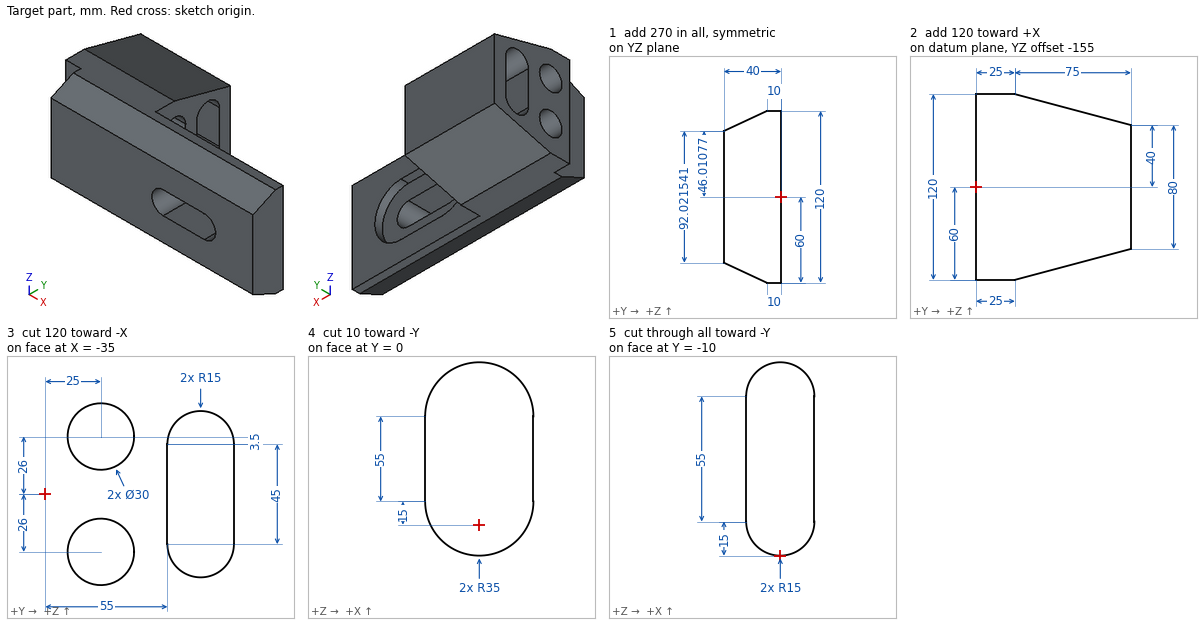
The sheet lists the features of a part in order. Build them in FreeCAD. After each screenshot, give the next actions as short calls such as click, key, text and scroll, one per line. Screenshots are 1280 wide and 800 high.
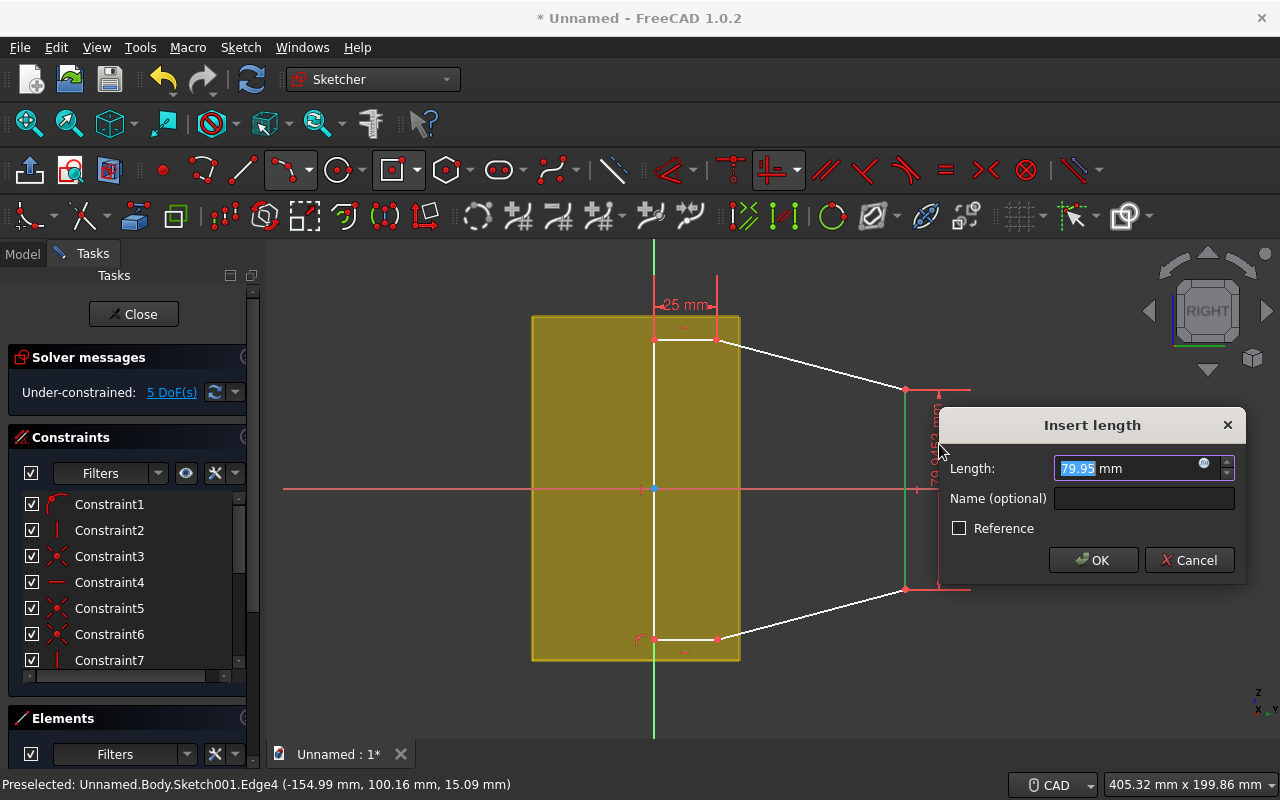
text(80)
key(Return)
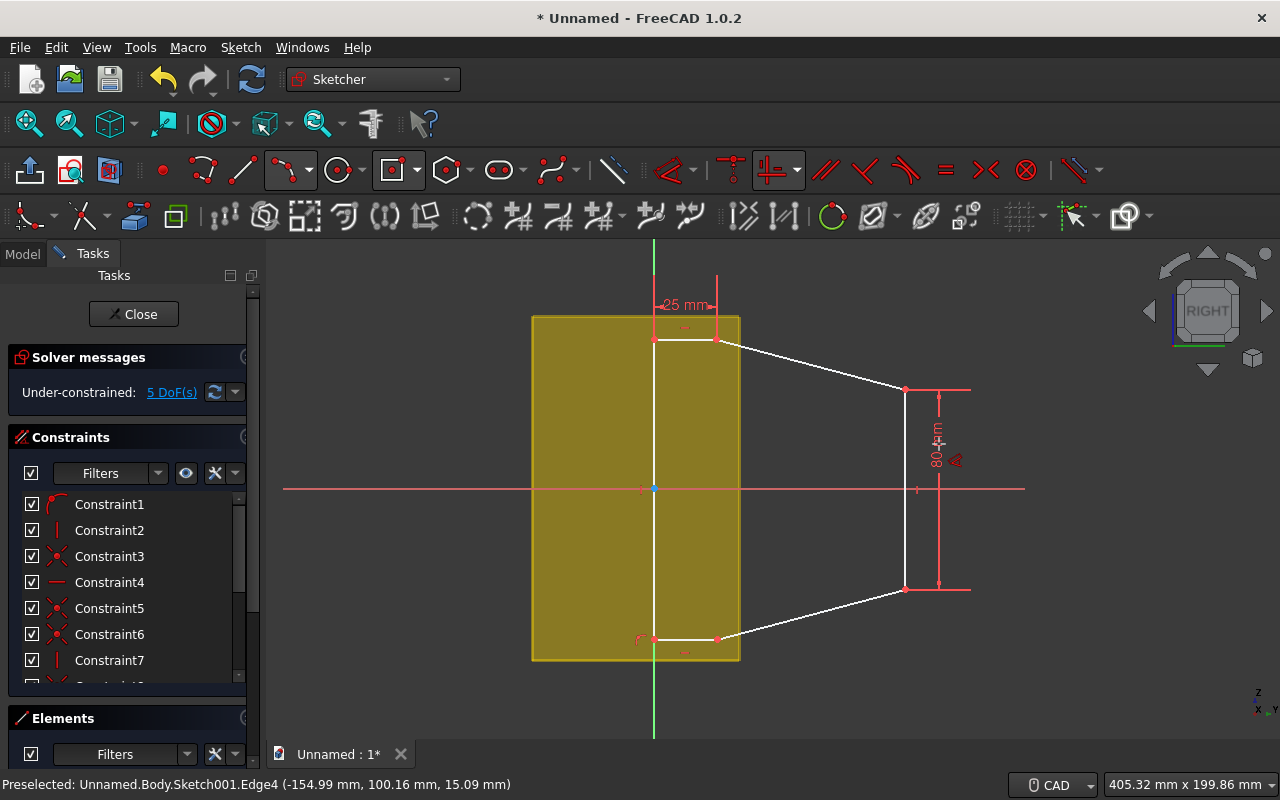
click(698, 640)
click(686, 674)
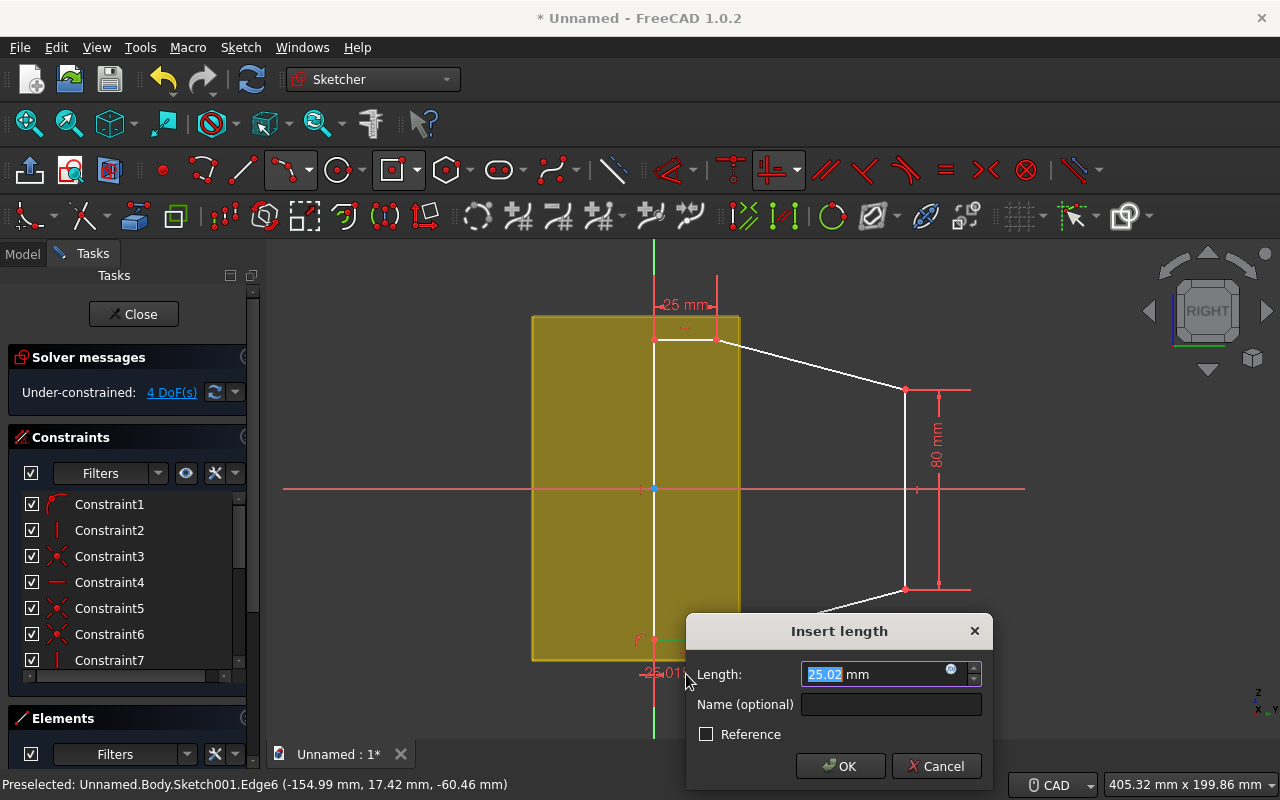
text(25)
key(Return)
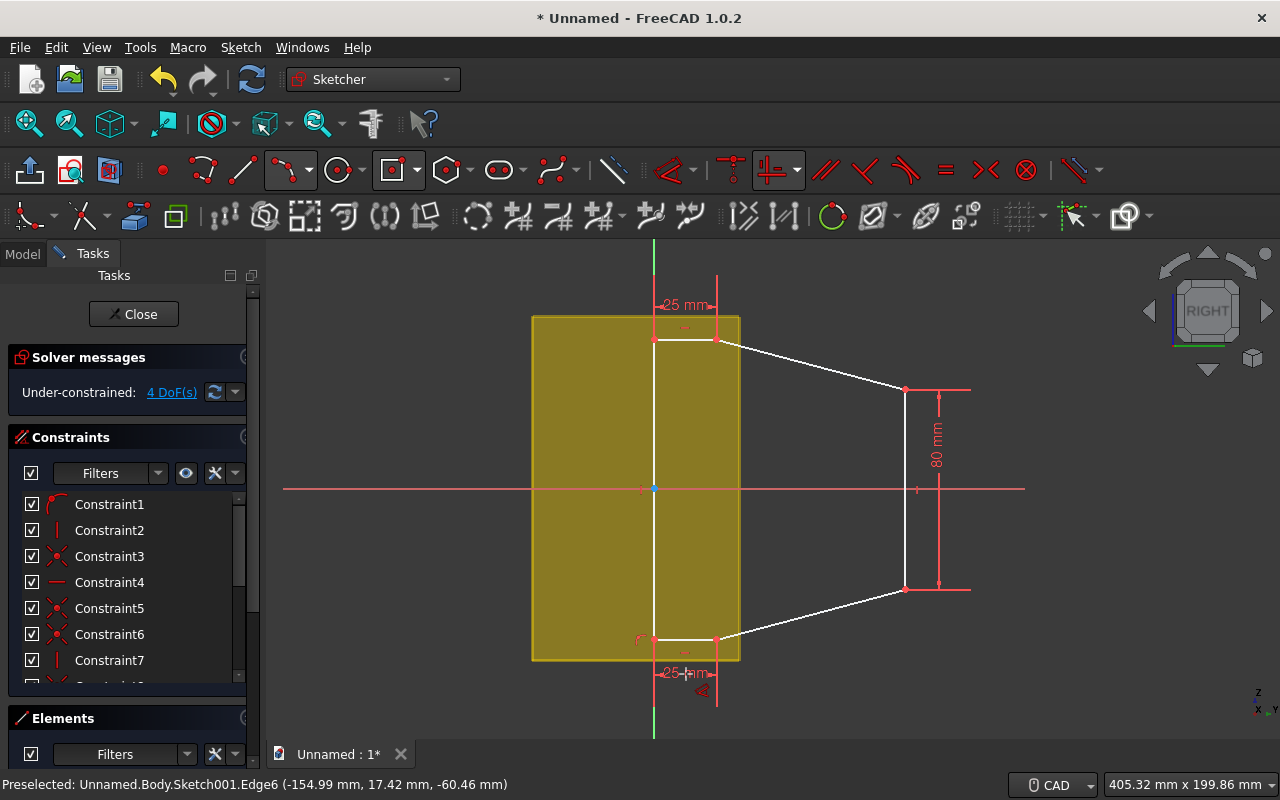
click(654, 550)
click(620, 421)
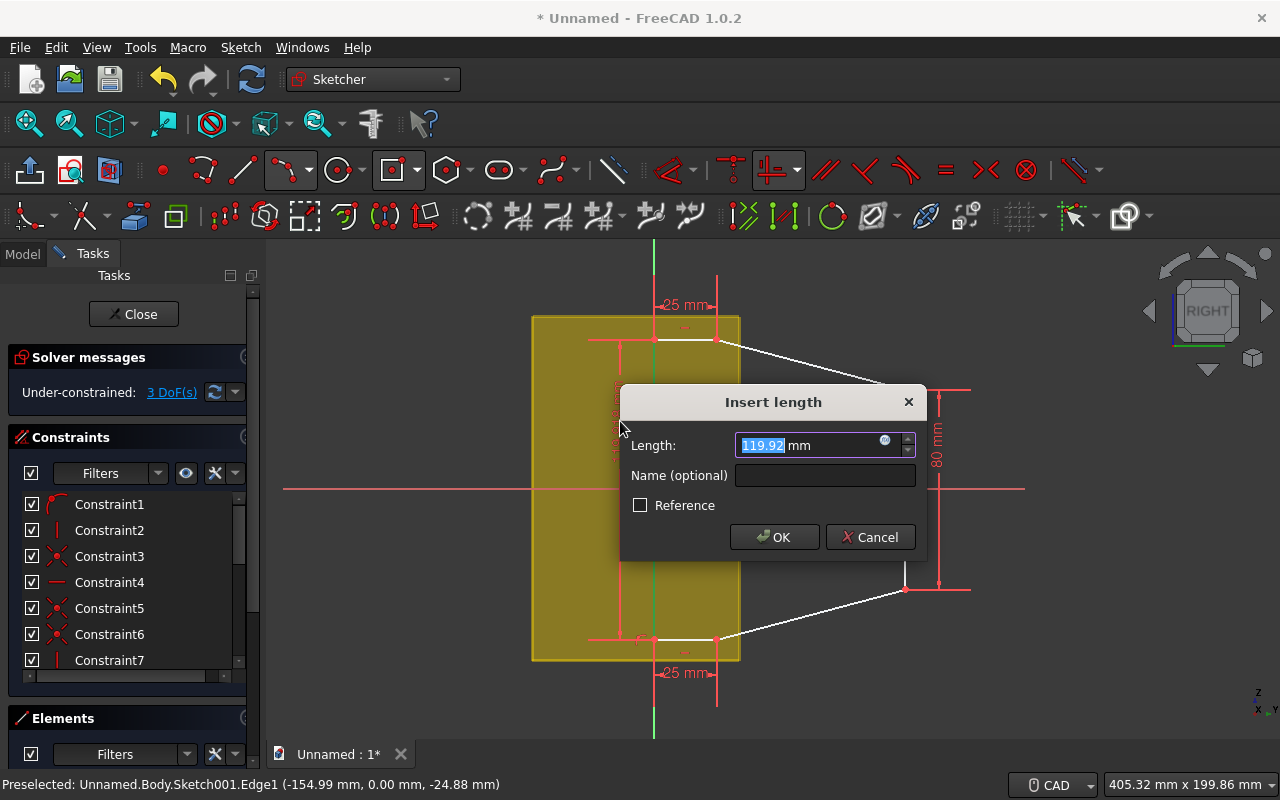
text(120)
key(Return)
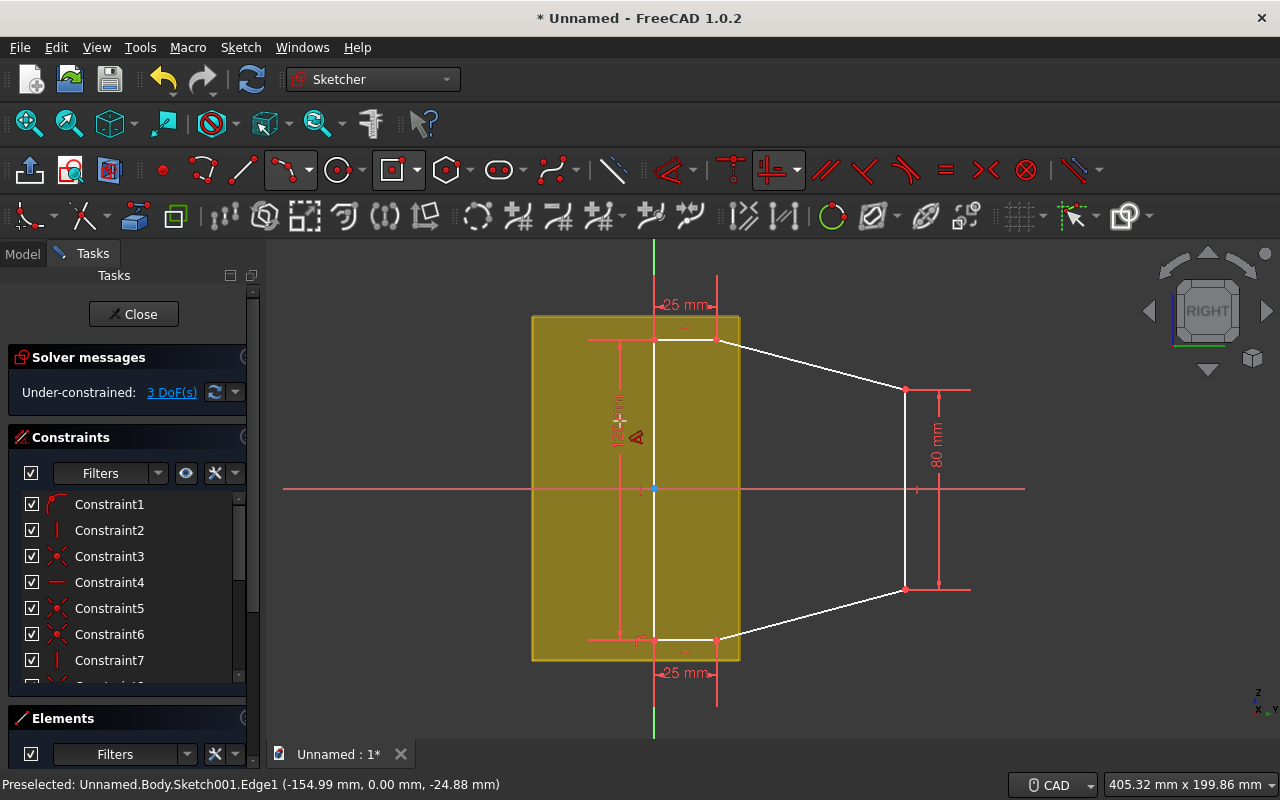
click(654, 640)
click(620, 564)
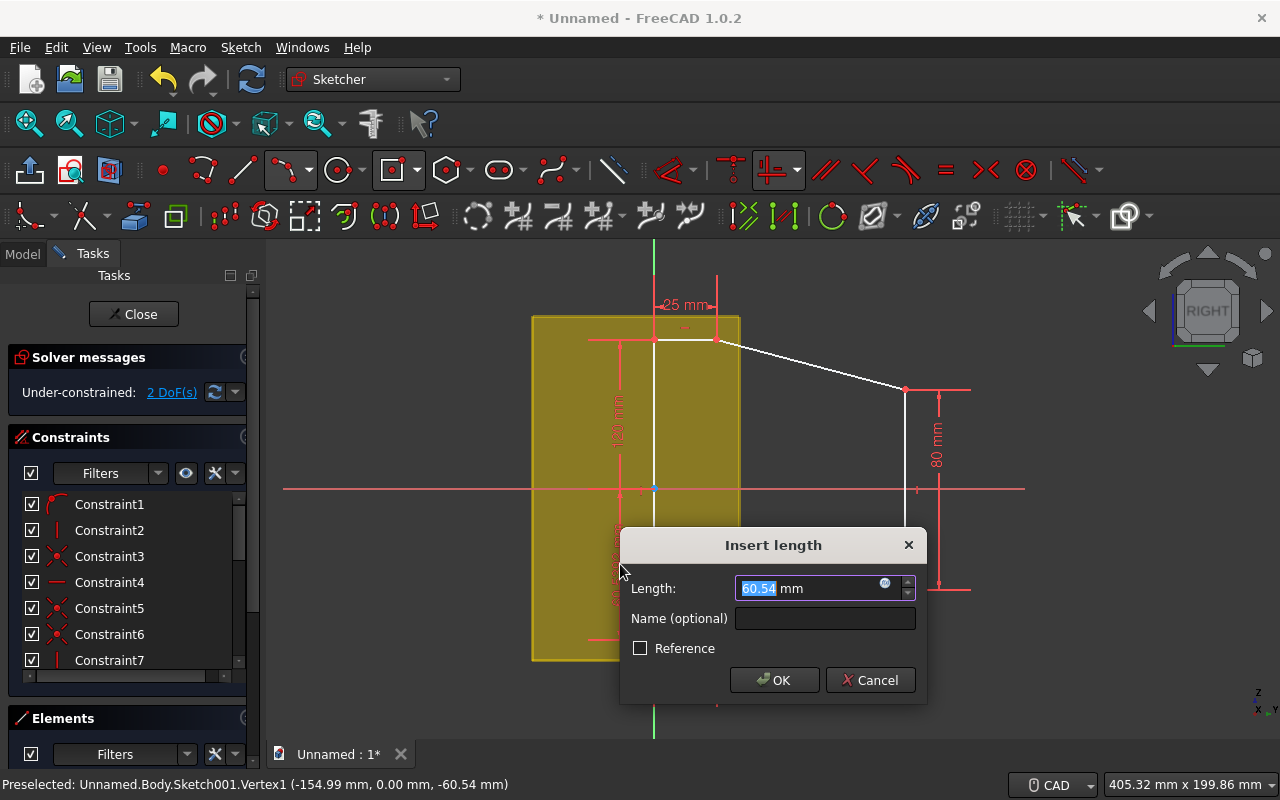
text(60)
key(Return)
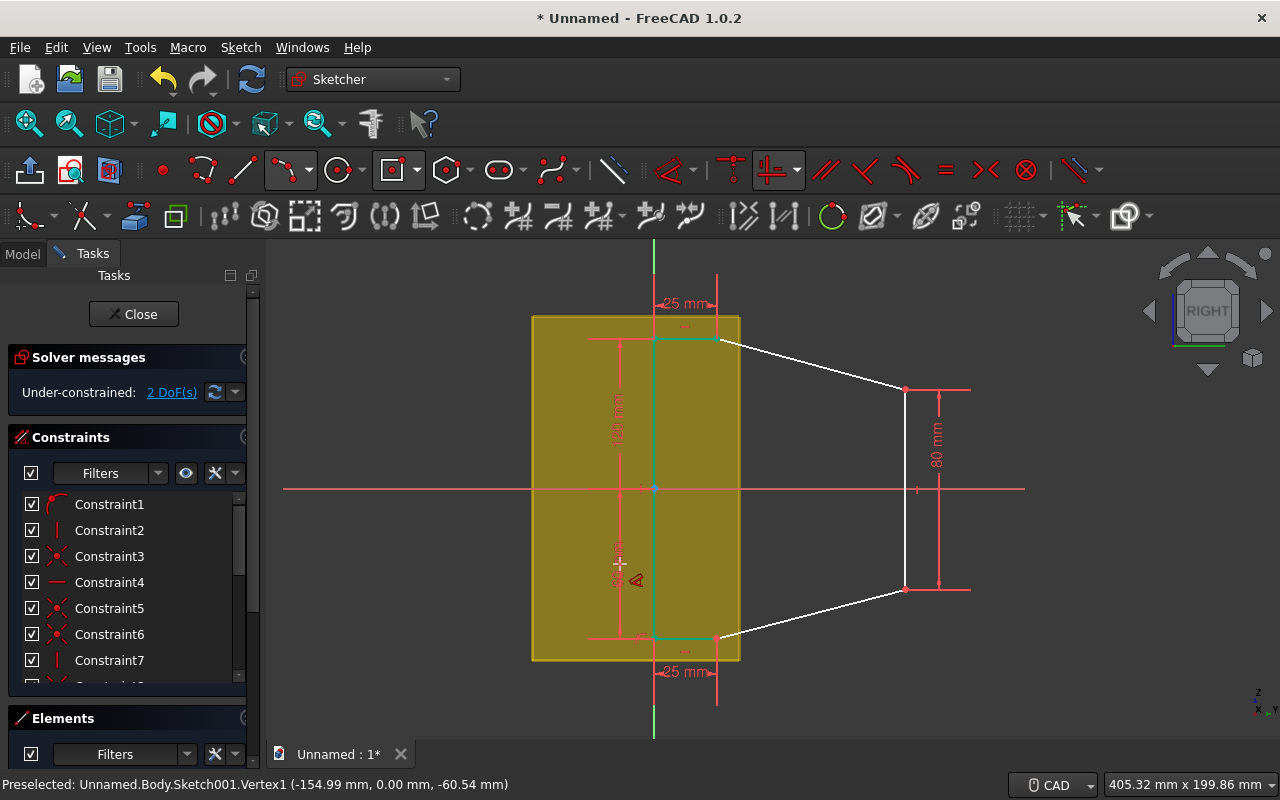
click(905, 390)
click(939, 417)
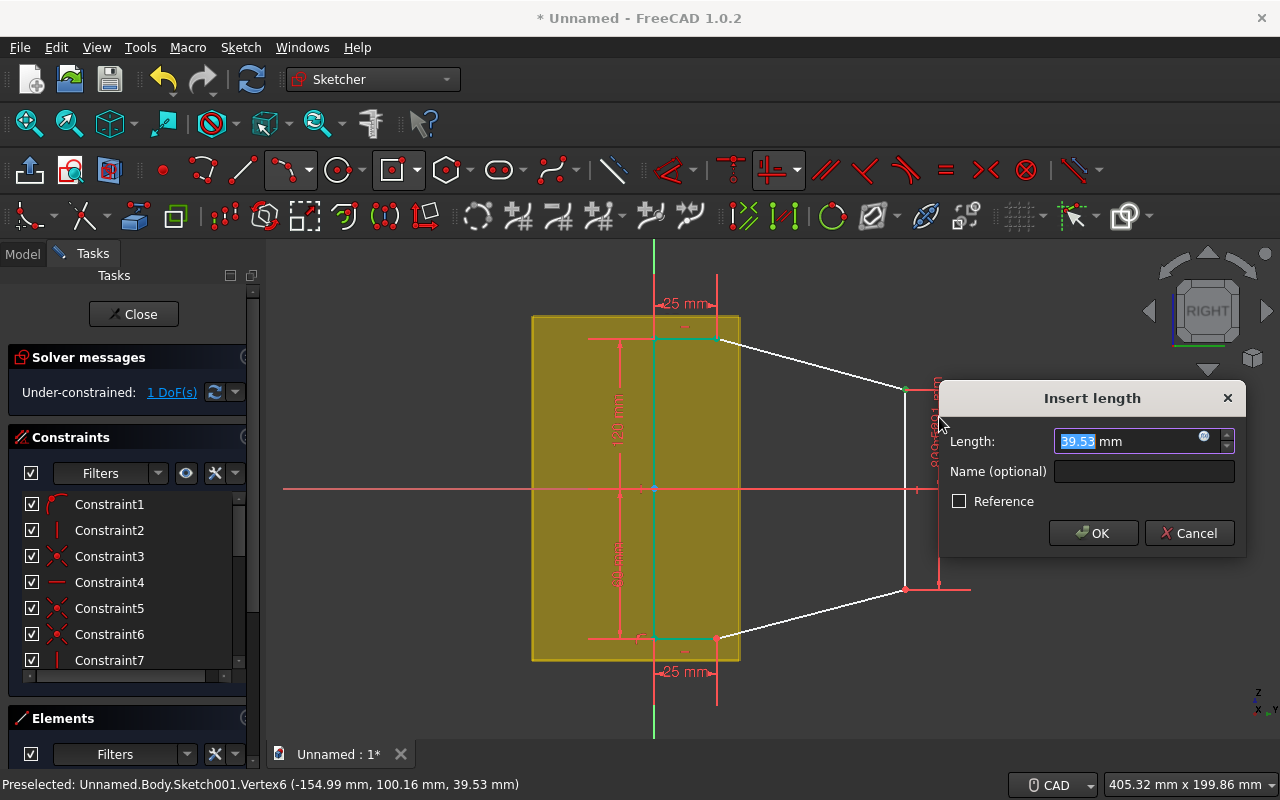
text(40)
key(Return)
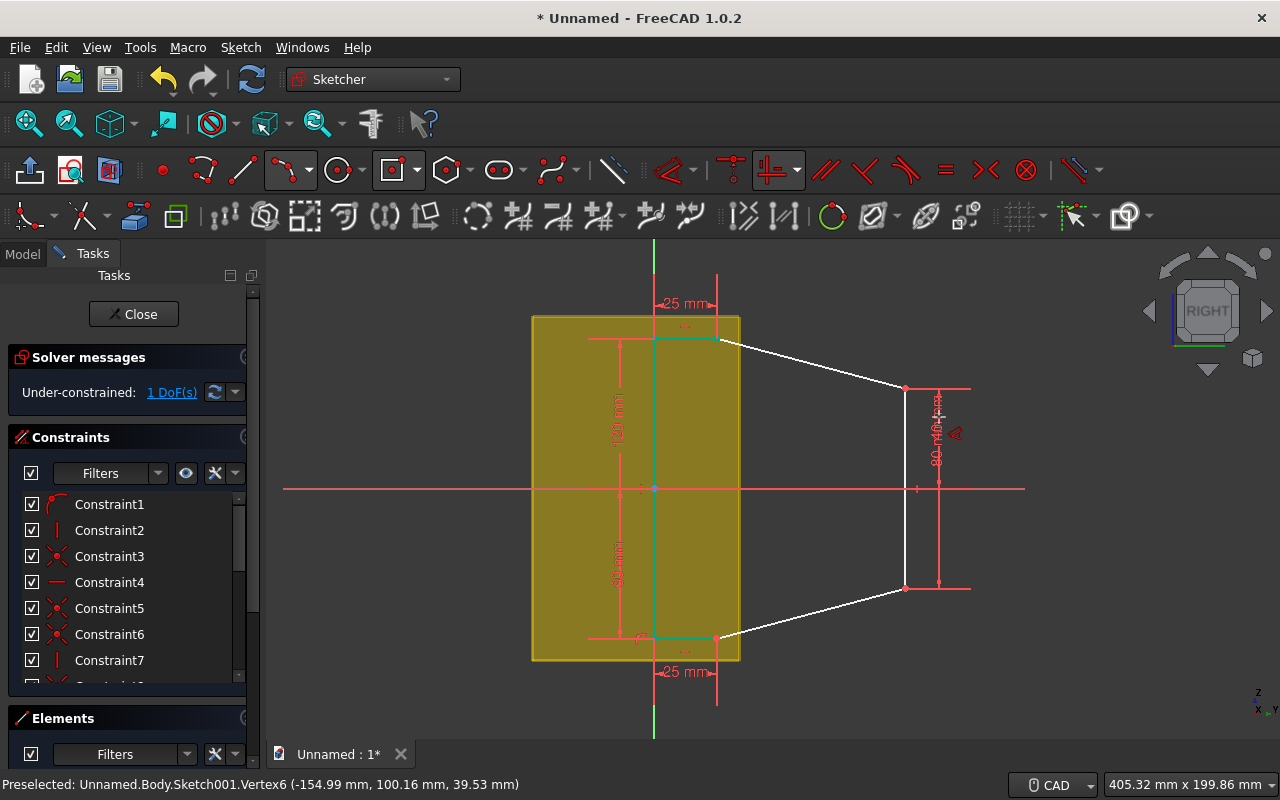
click(773, 354)
click(811, 305)